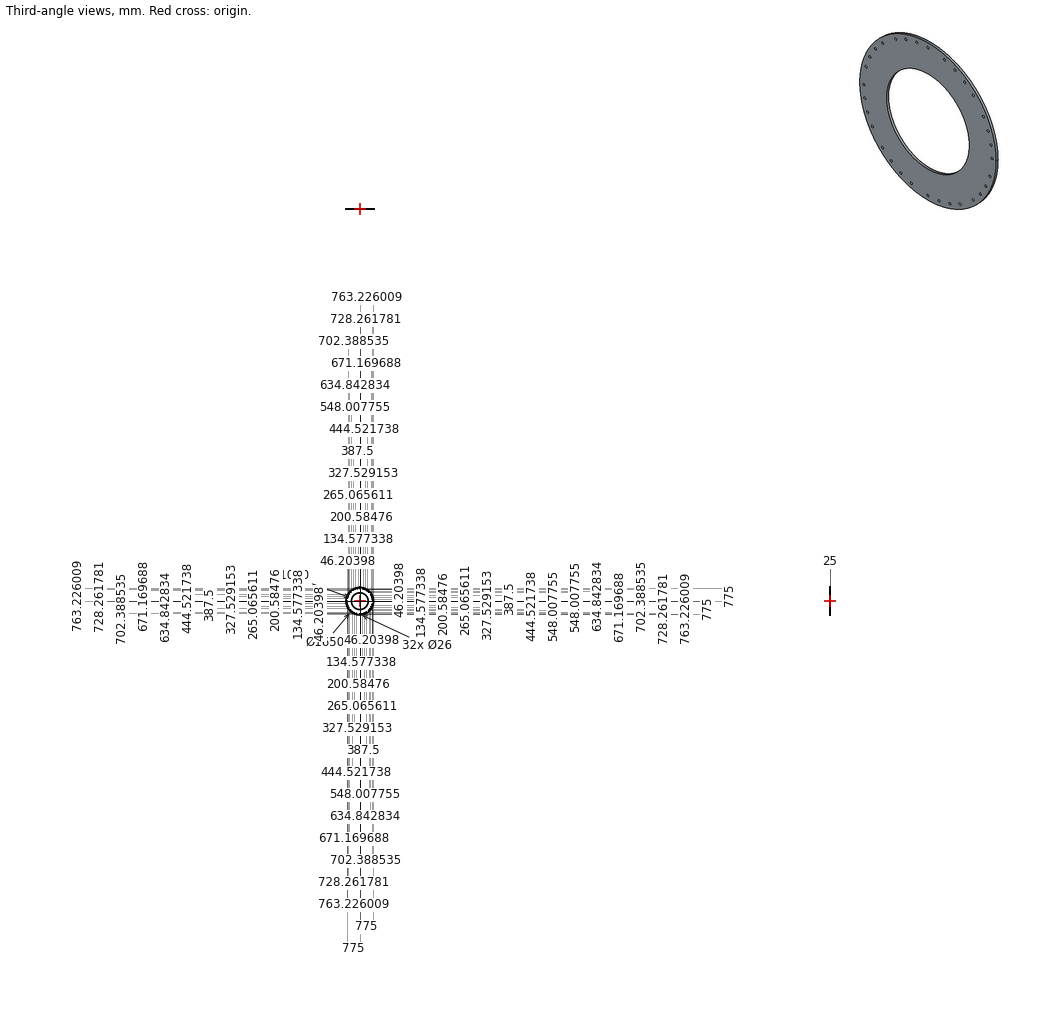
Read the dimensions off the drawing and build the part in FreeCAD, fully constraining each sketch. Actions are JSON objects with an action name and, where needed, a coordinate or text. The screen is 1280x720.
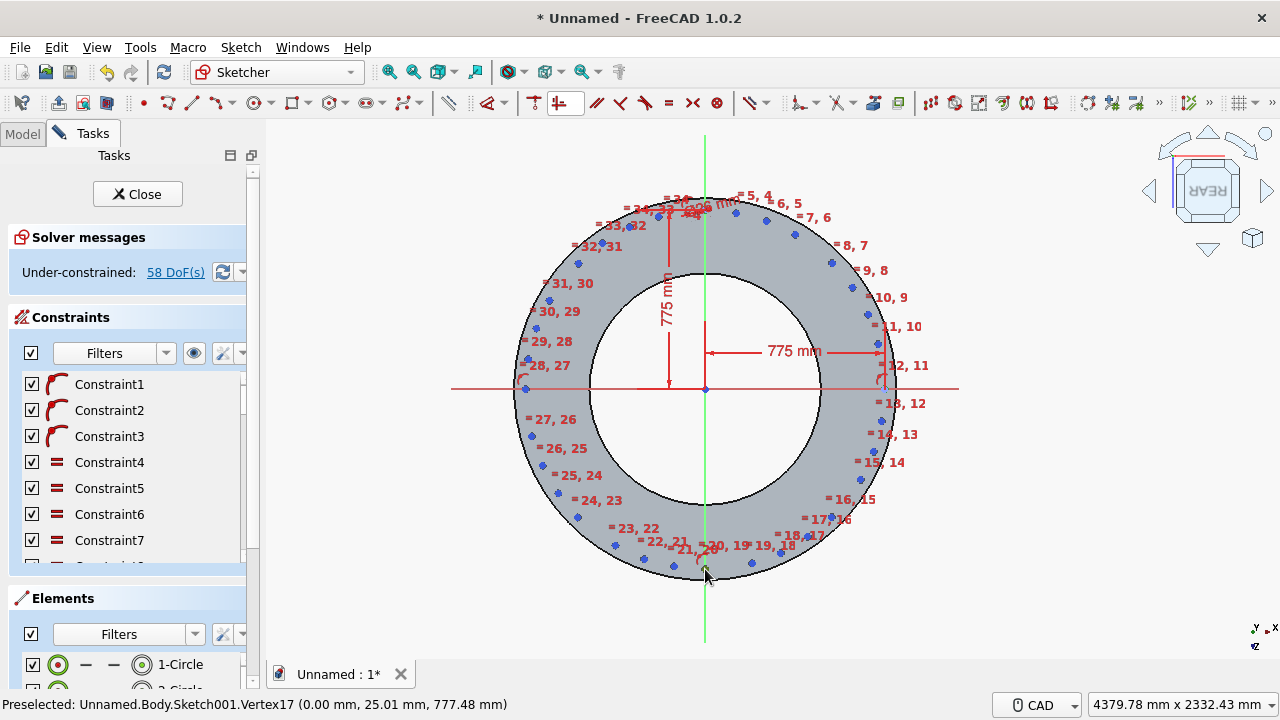
{"action": "key", "text": "i"}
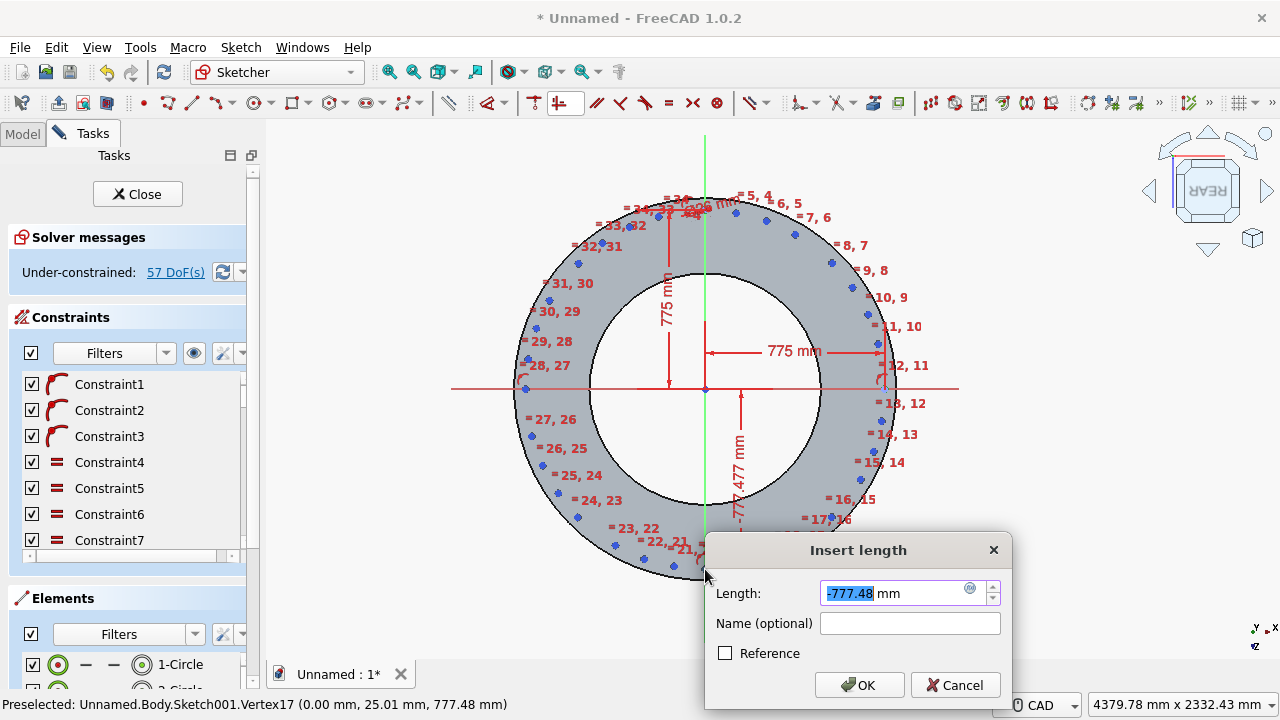
{"action": "type", "text": "-775"}
{"action": "key", "text": "Return"}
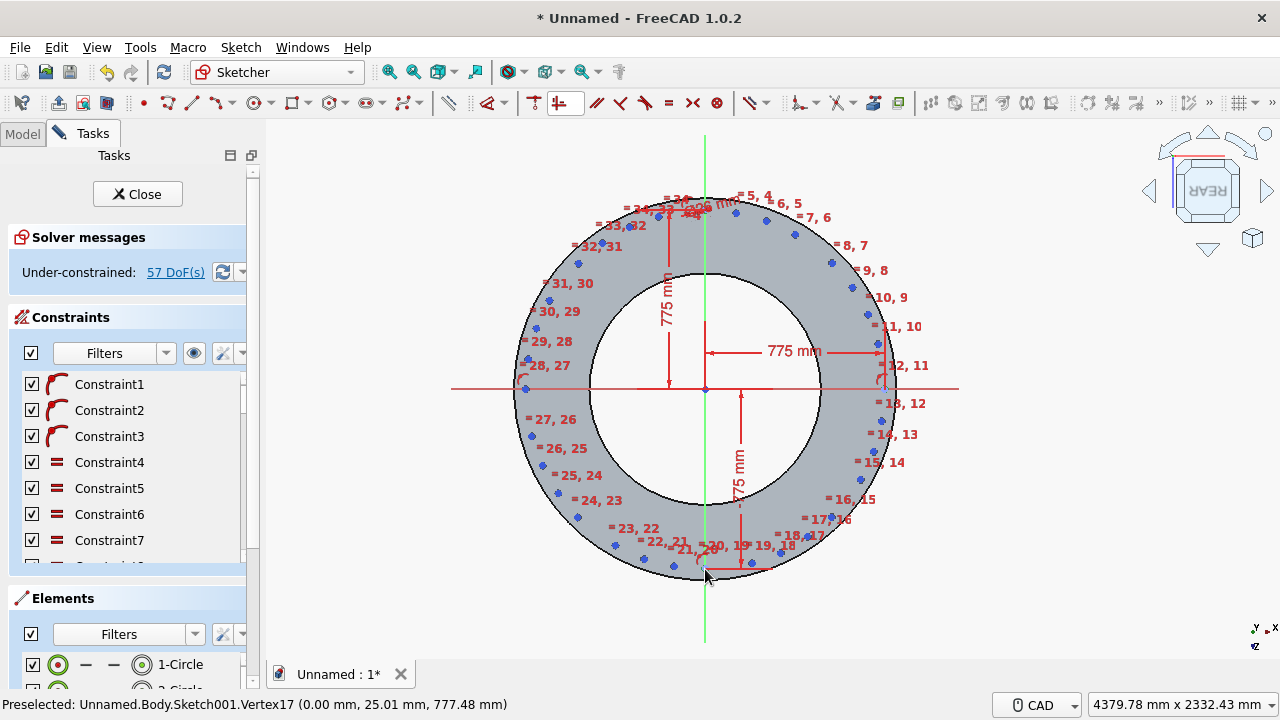
{"action": "left_click", "coordinate": [526, 389]}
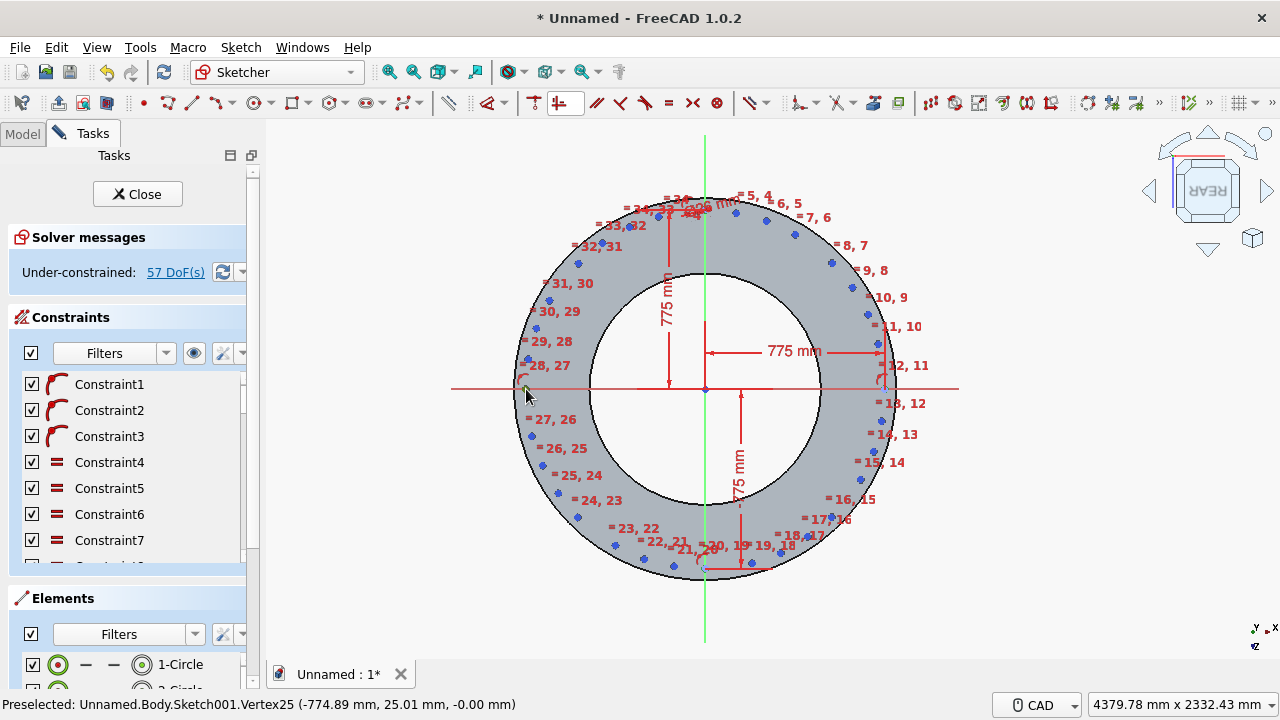
{"action": "key", "text": "l"}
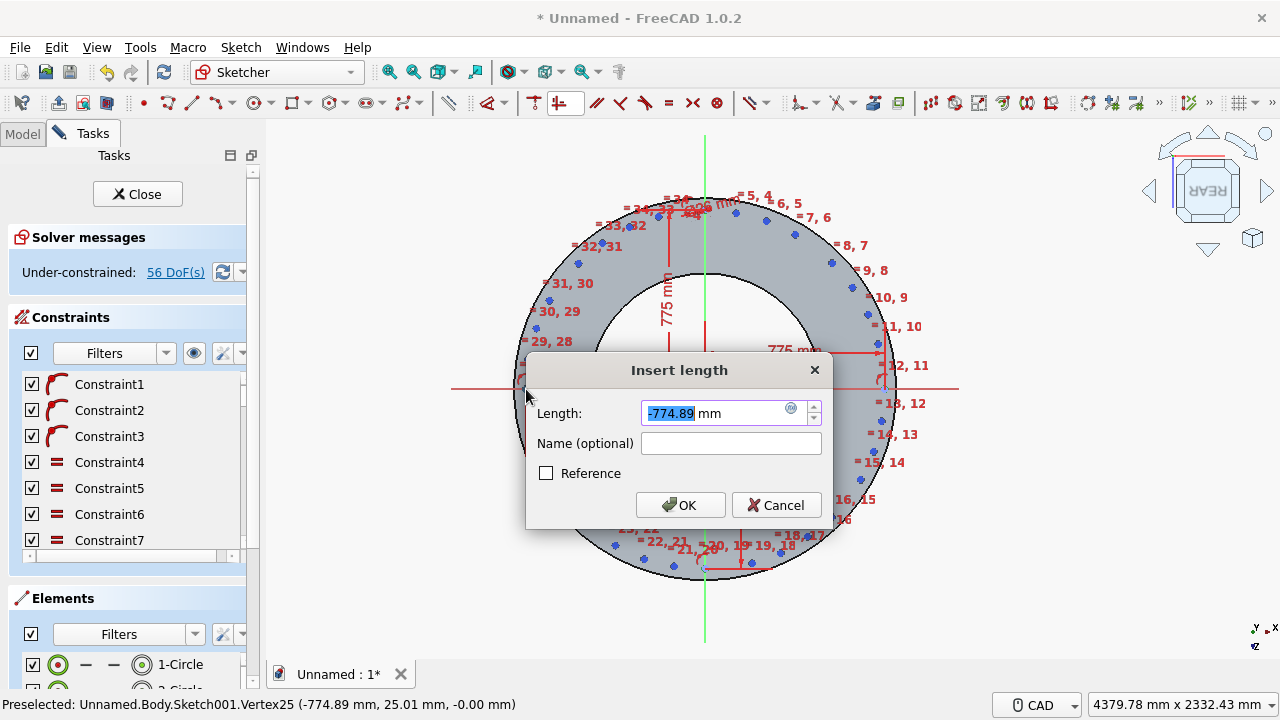
{"action": "type", "text": "-775"}
{"action": "key", "text": "Return"}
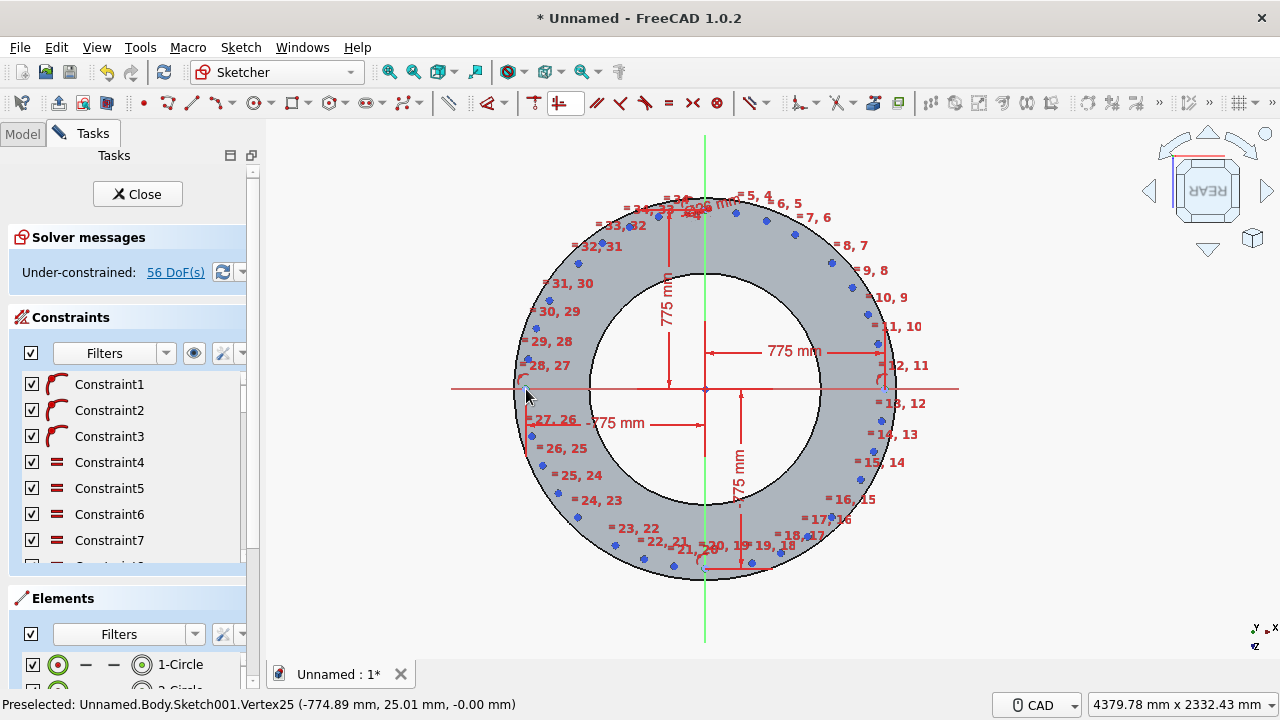
{"action": "left_click", "coordinate": [795, 235]}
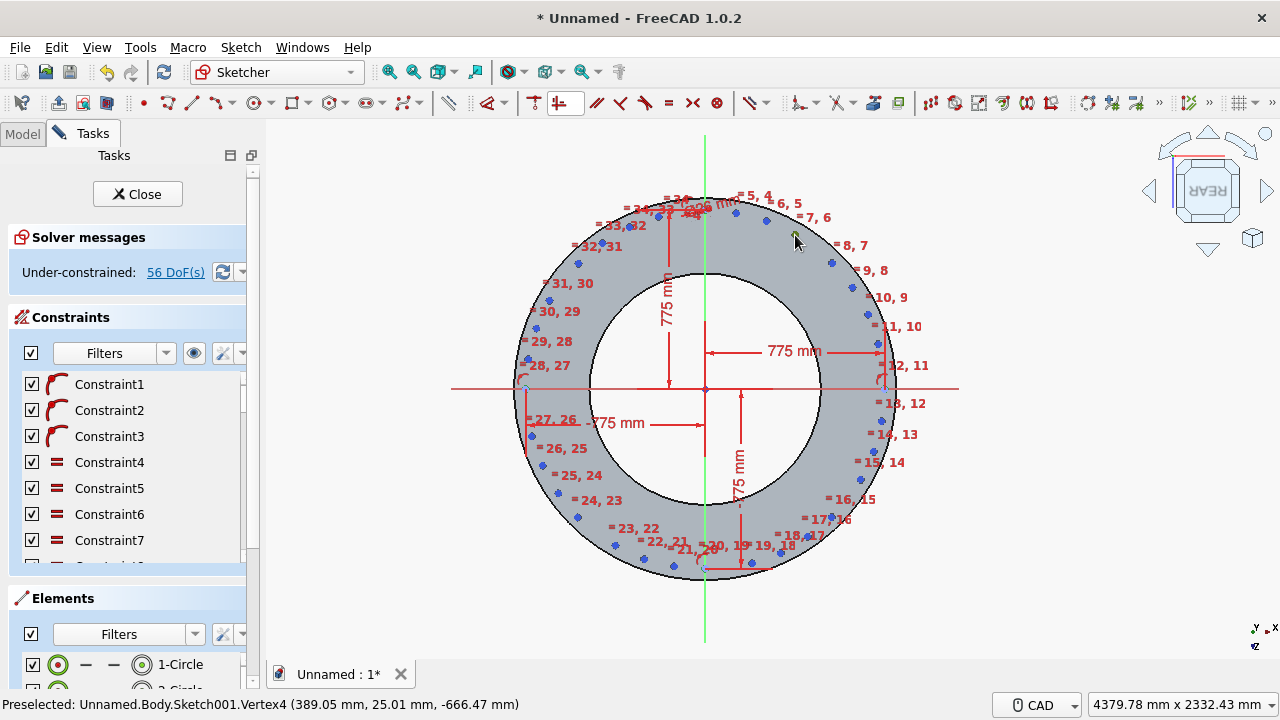
{"action": "key", "text": "l"}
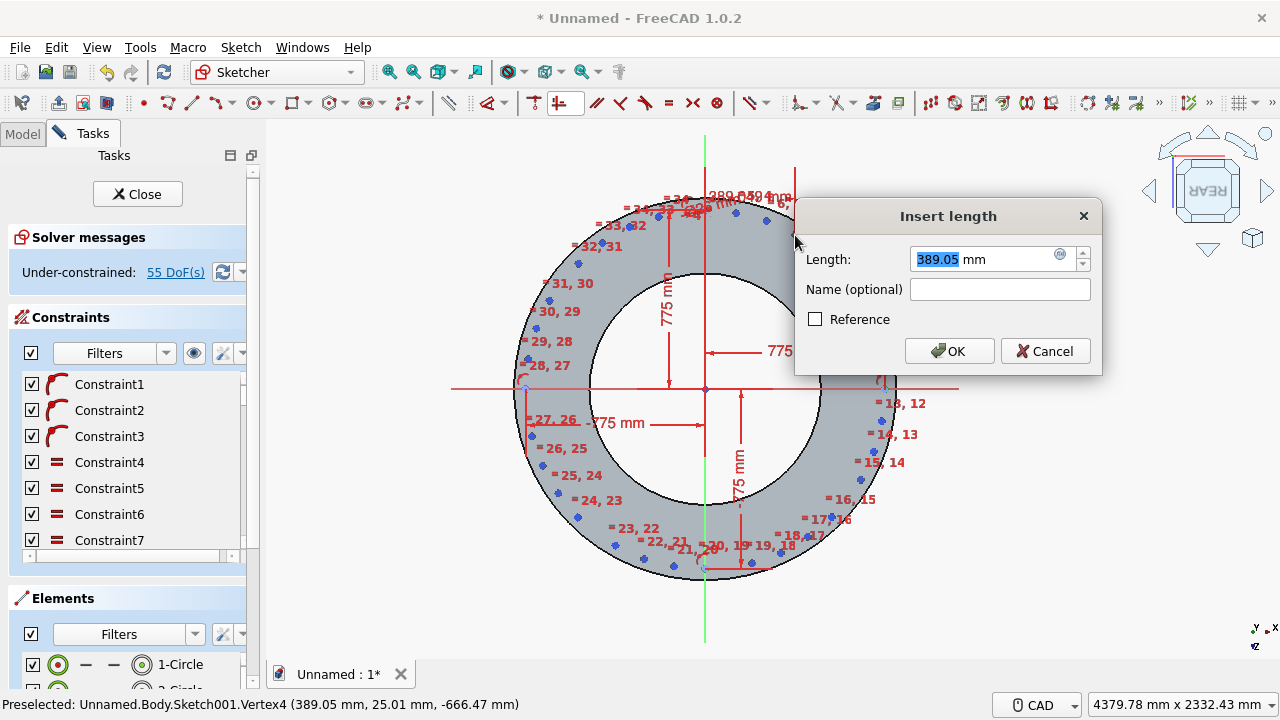
{"action": "type", "text": "387.5"}
{"action": "key", "text": "Return"}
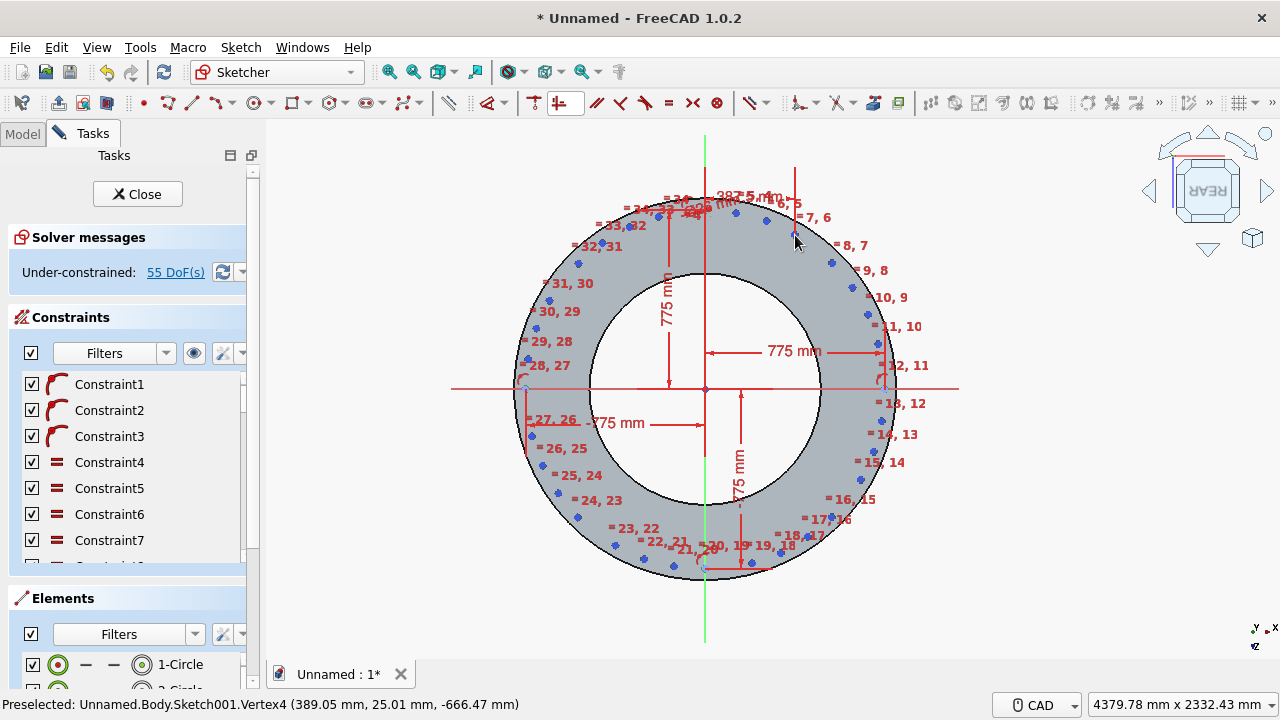
{"action": "left_click", "coordinate": [861, 480]}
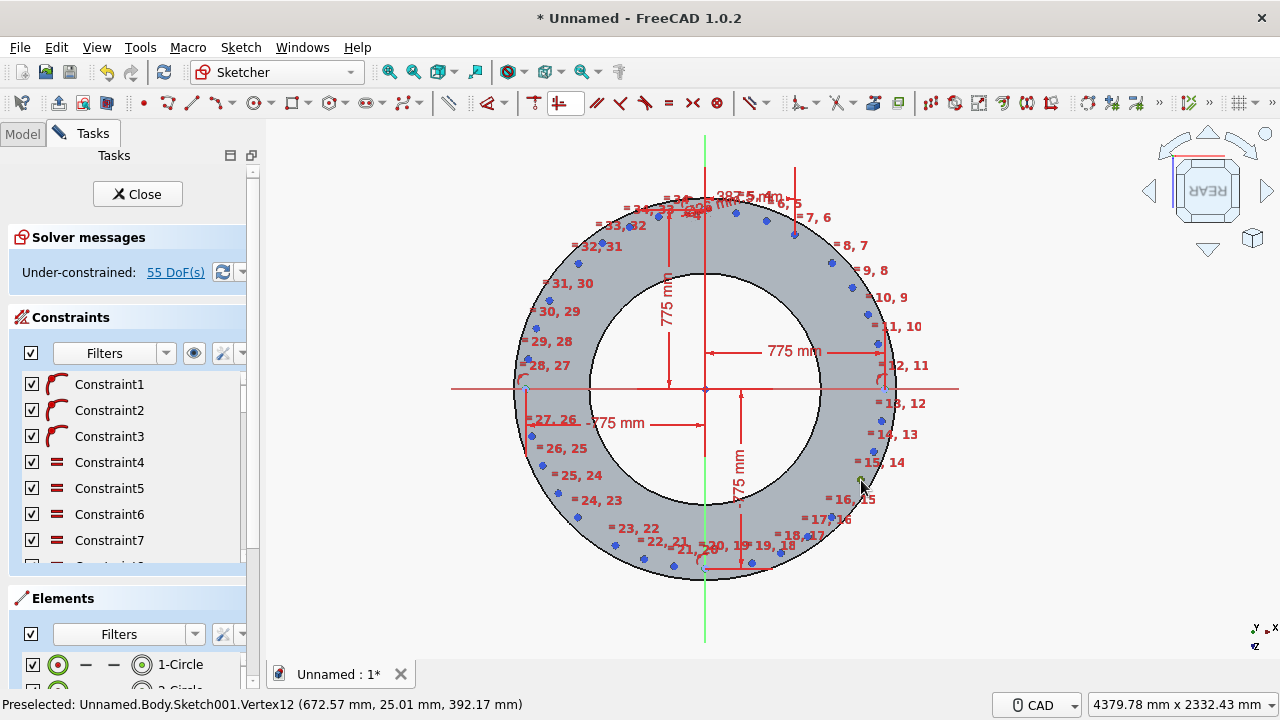
{"action": "key", "text": "i"}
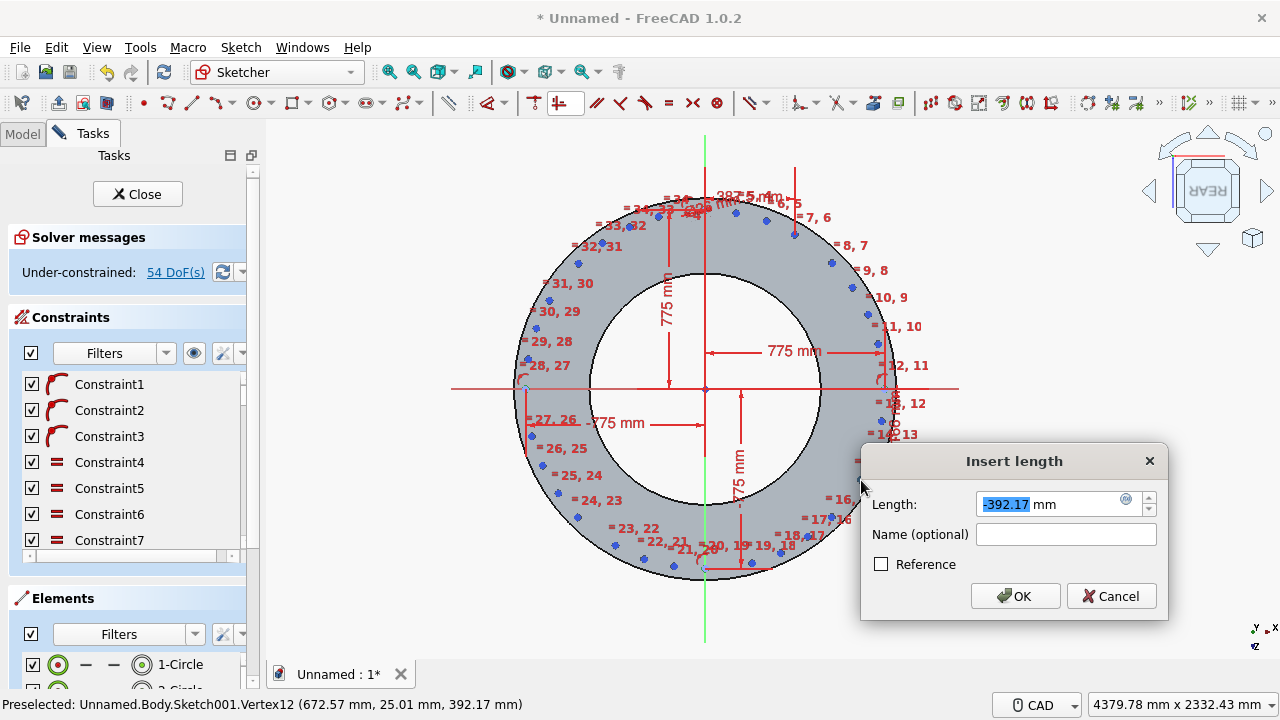
{"action": "type", "text": "-387.5"}
{"action": "key", "text": "Return"}